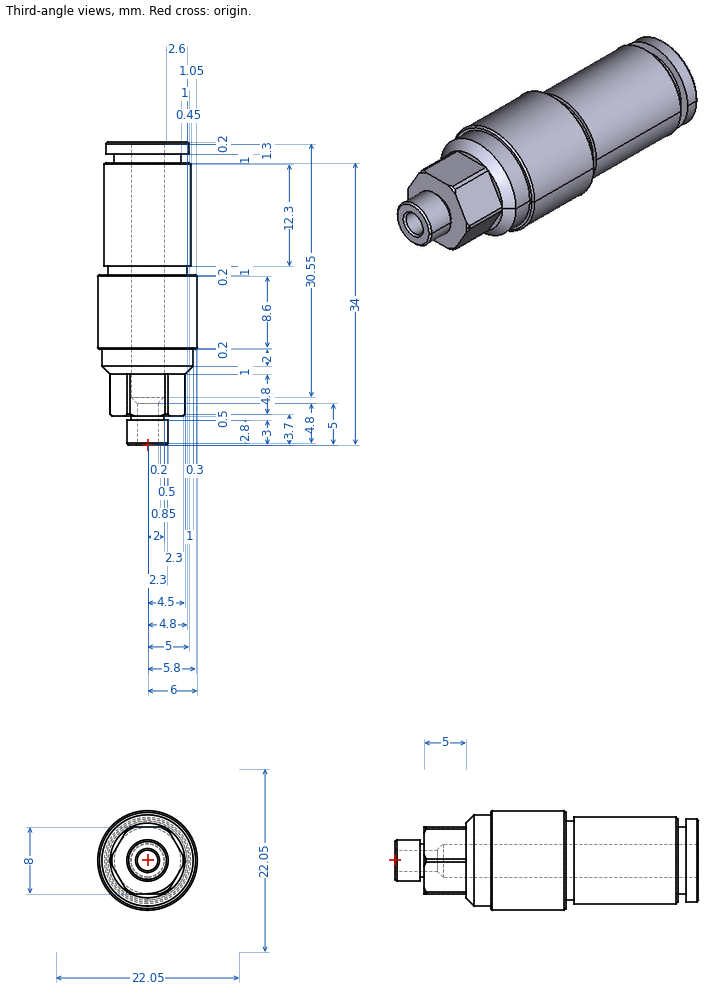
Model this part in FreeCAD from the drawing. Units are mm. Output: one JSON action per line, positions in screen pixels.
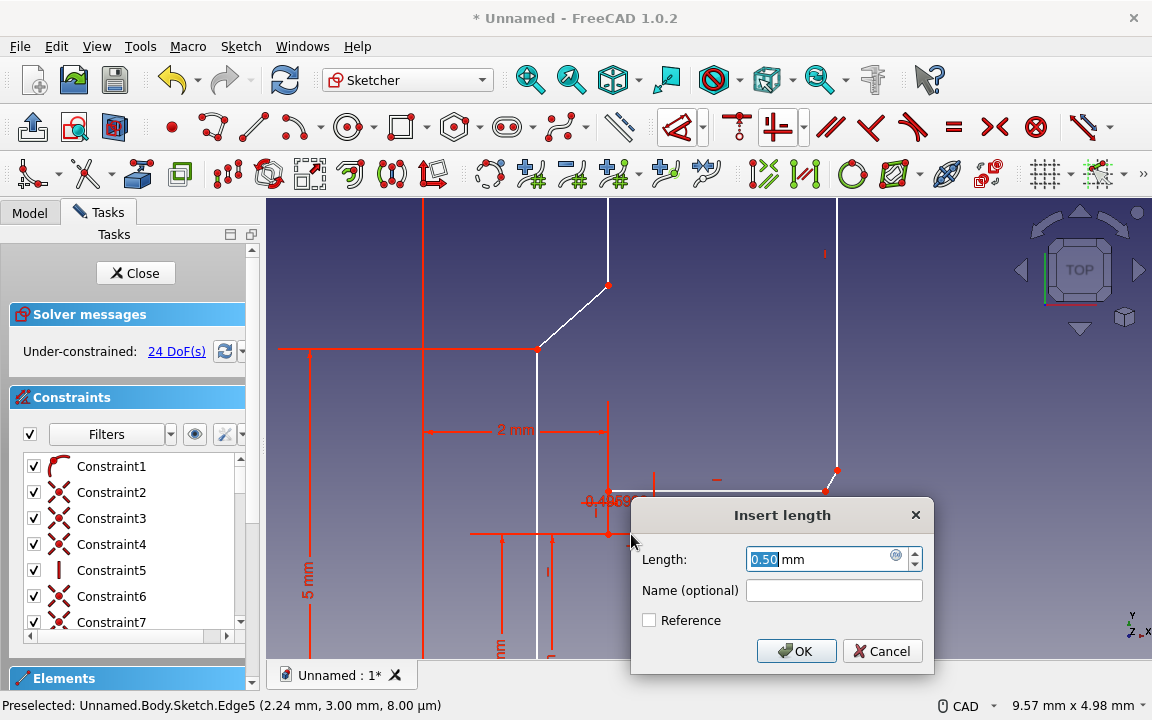
{"action": "type", "text": "0.5"}
{"action": "key", "text": "Return"}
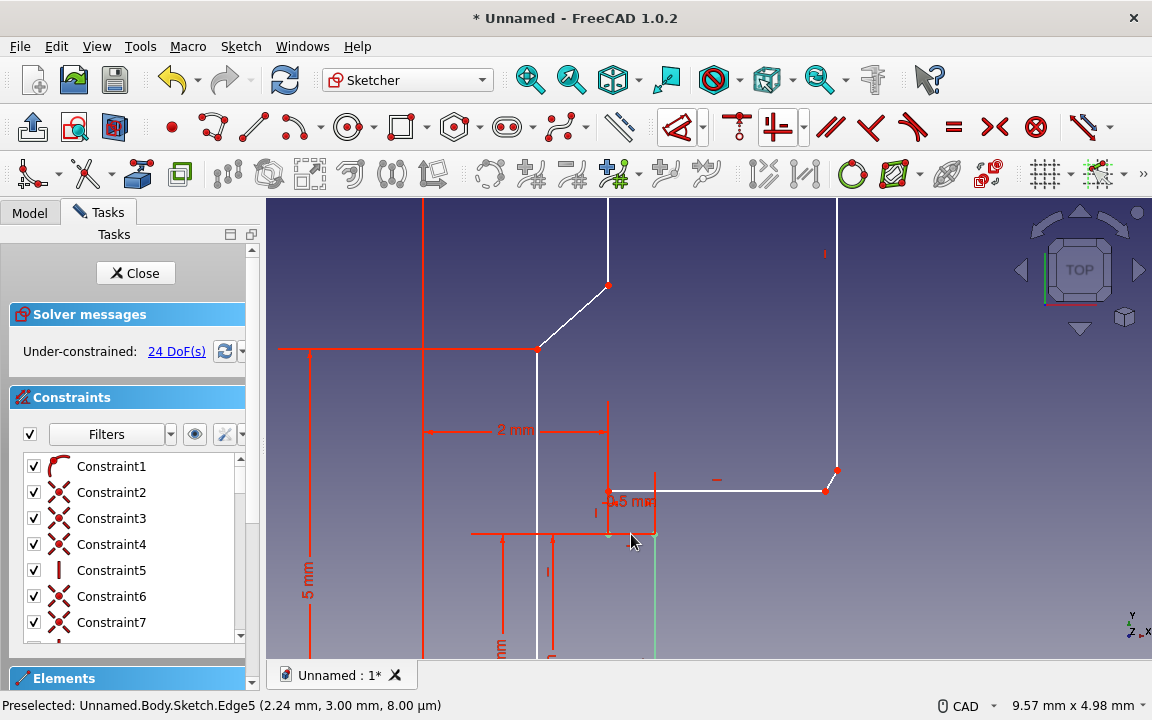
{"action": "left_click", "coordinate": [608, 521]}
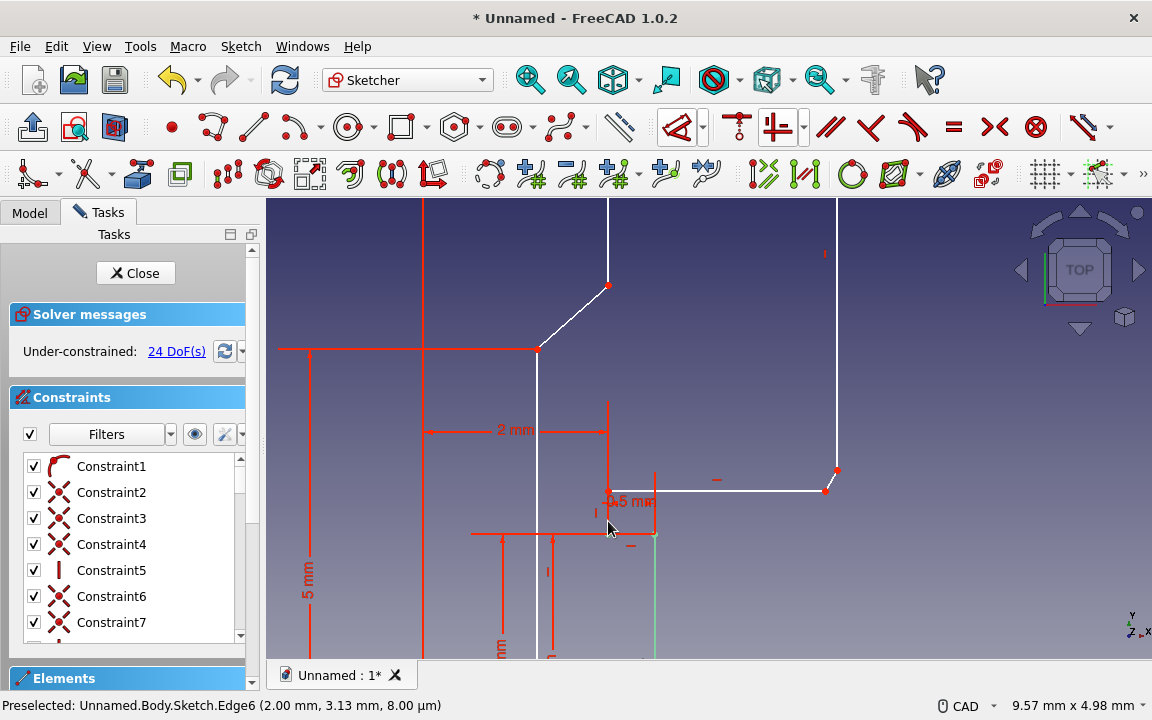
{"action": "left_click", "coordinate": [702, 128]}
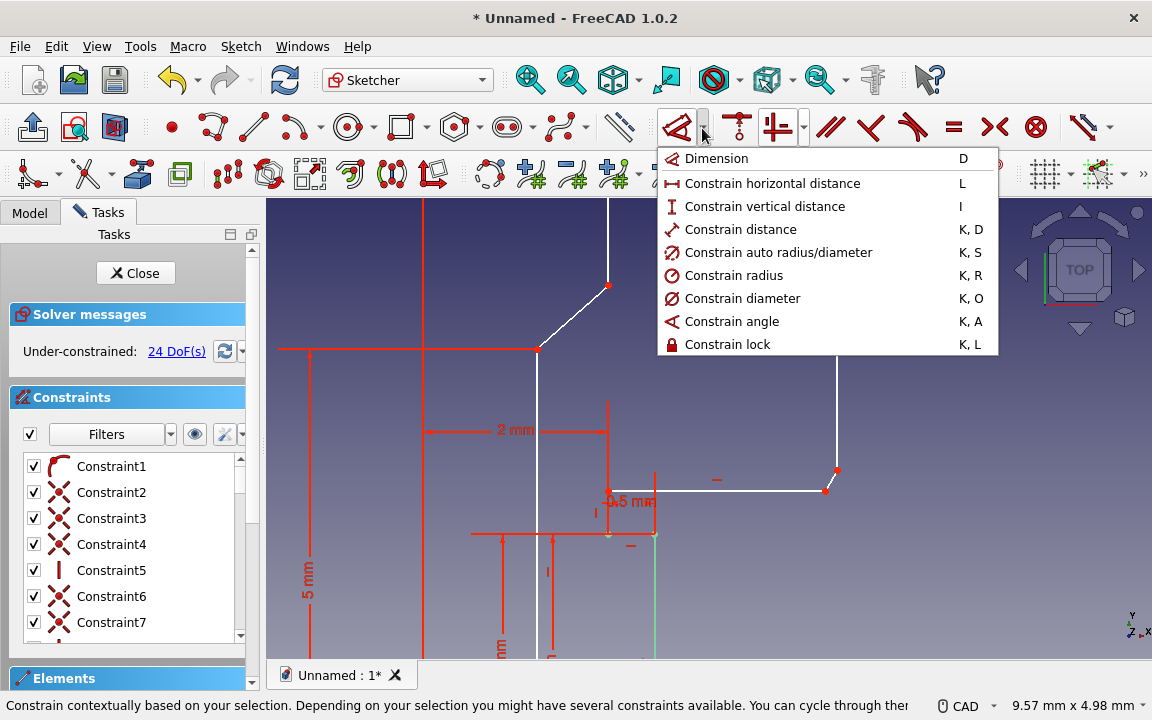
{"action": "left_click", "coordinate": [828, 206]}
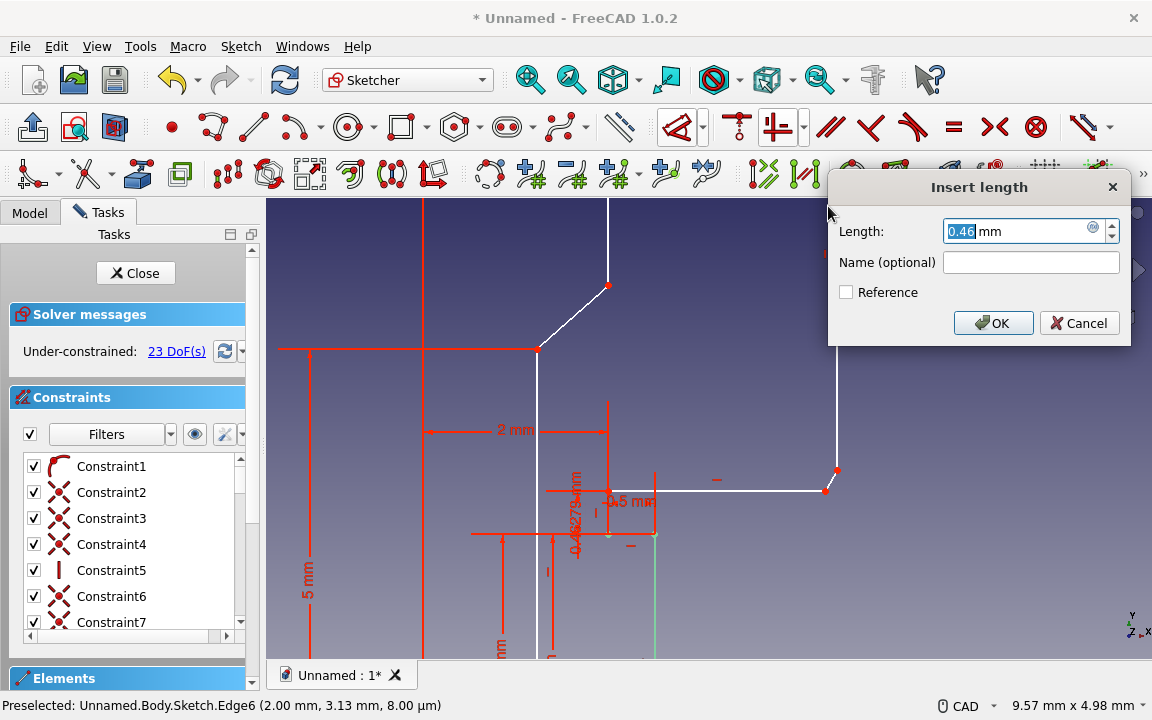
{"action": "type", "text": "0.5"}
{"action": "key", "text": "Return"}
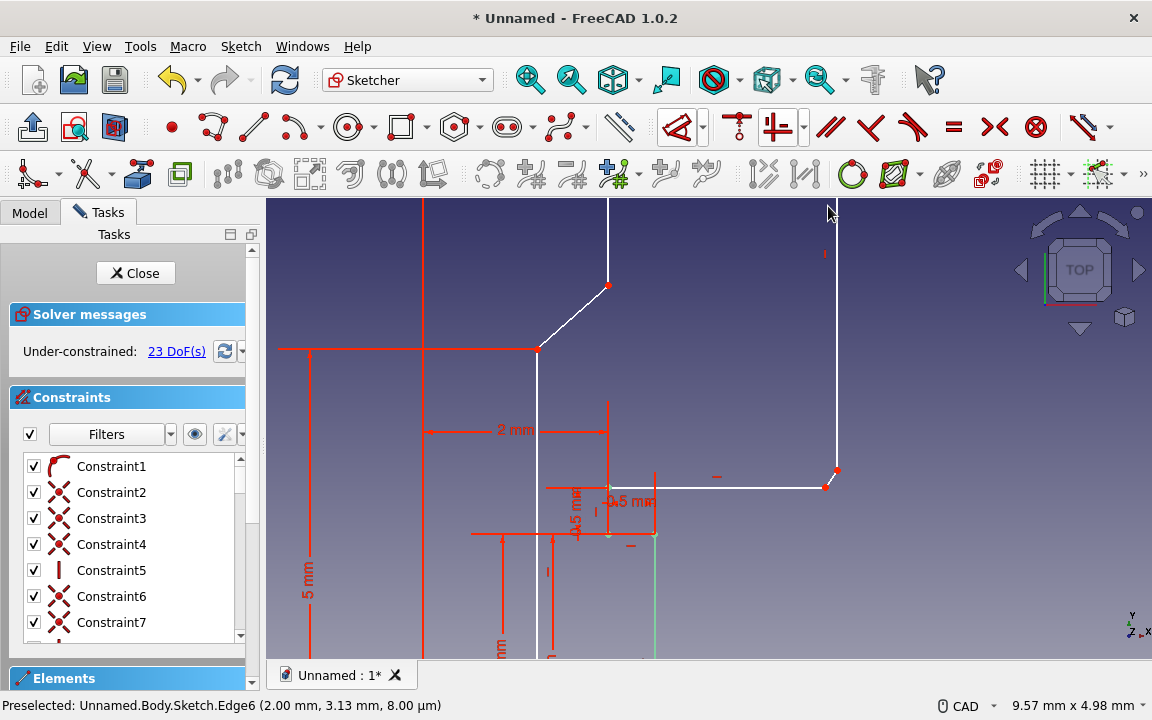
{"action": "scroll", "coordinate": [634, 559], "scroll_direction": "down", "scroll_amount": 12}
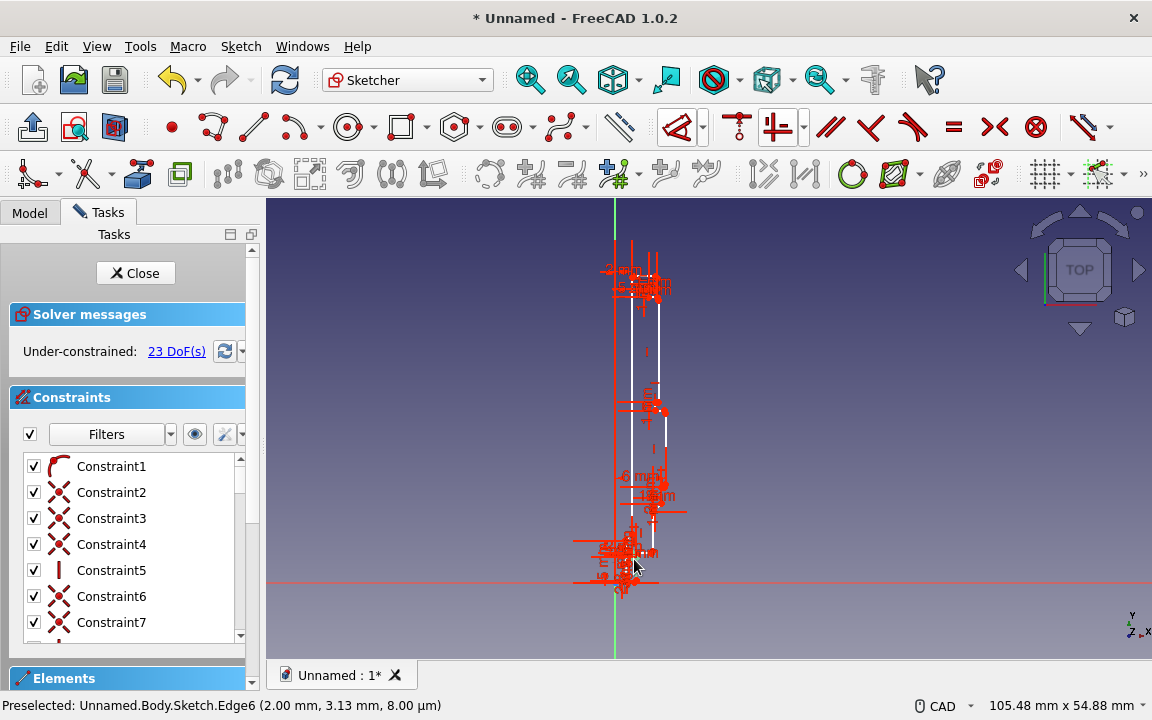
{"action": "scroll", "coordinate": [638, 553], "scroll_direction": "up", "scroll_amount": 6}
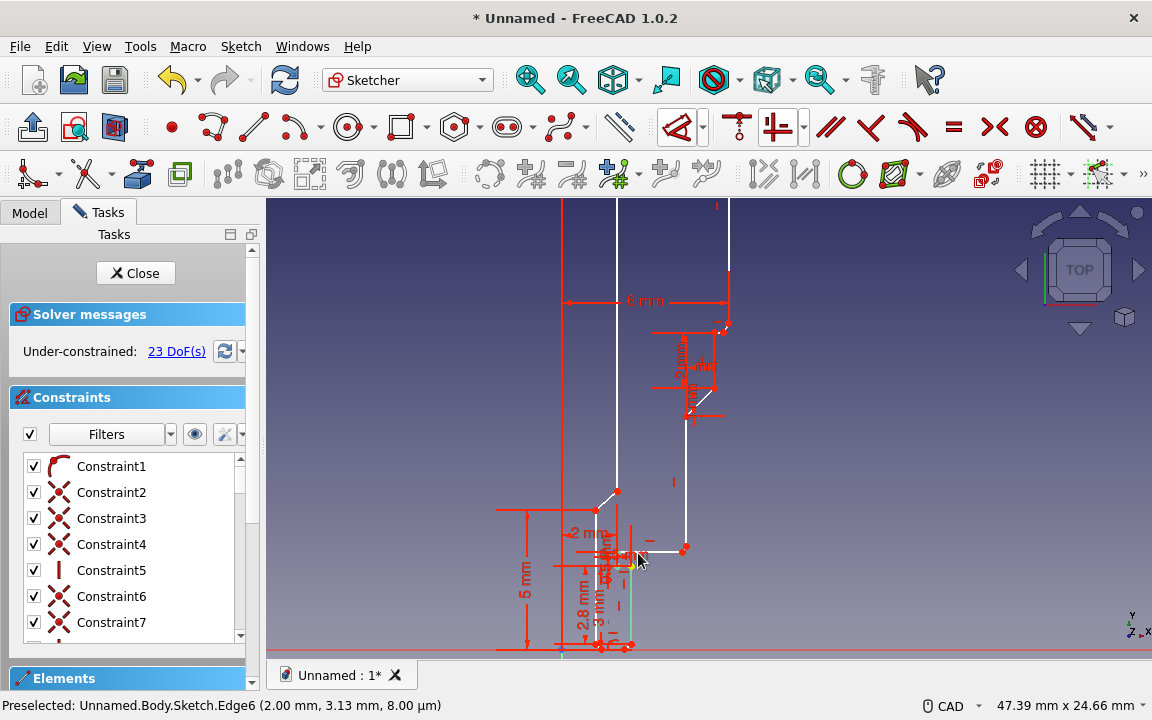
{"action": "left_click", "coordinate": [663, 552]}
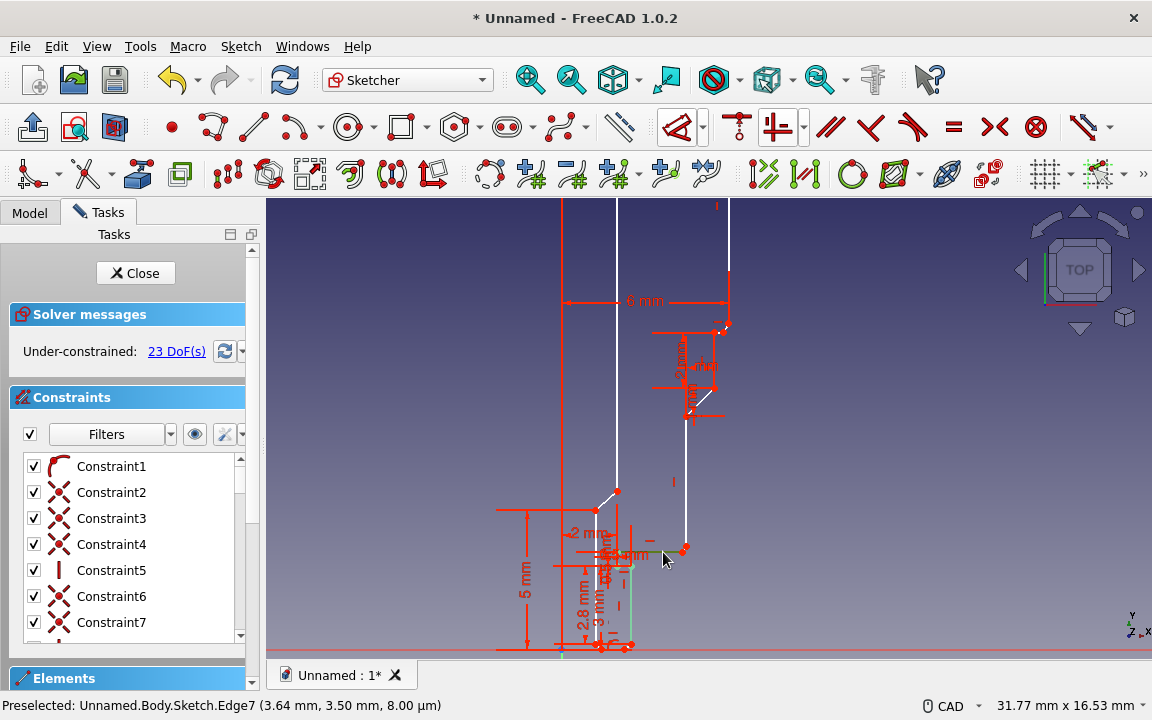
{"action": "left_click", "coordinate": [702, 128]}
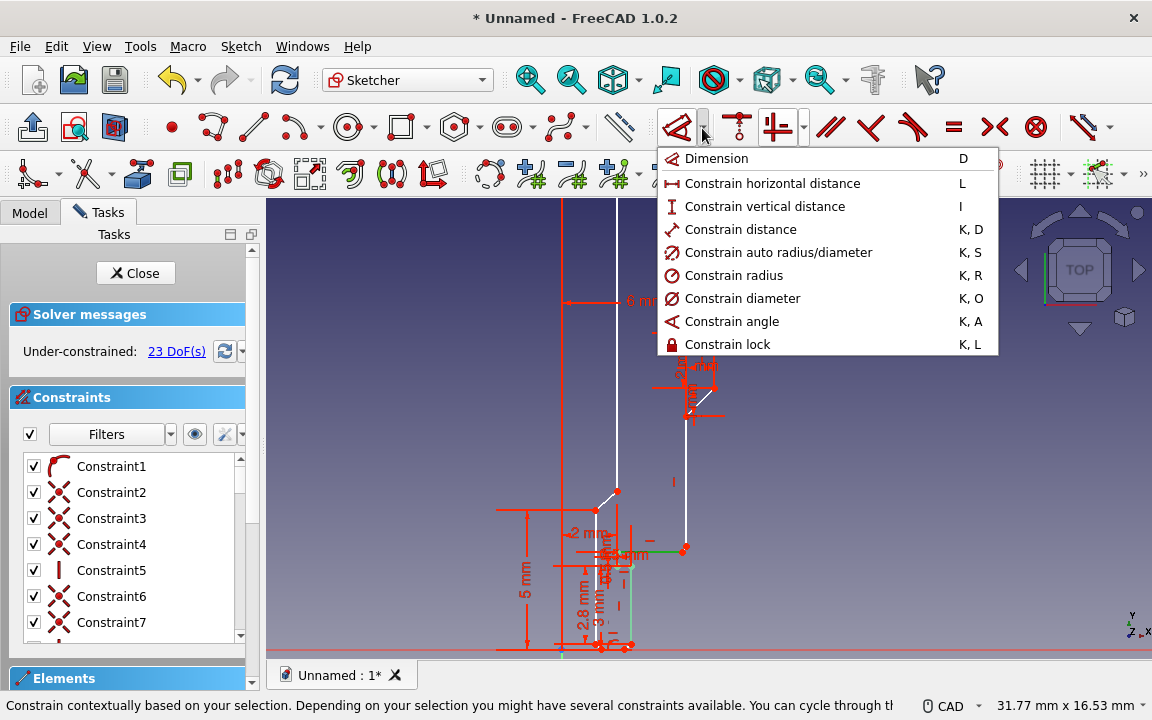
{"action": "left_click", "coordinate": [828, 184]}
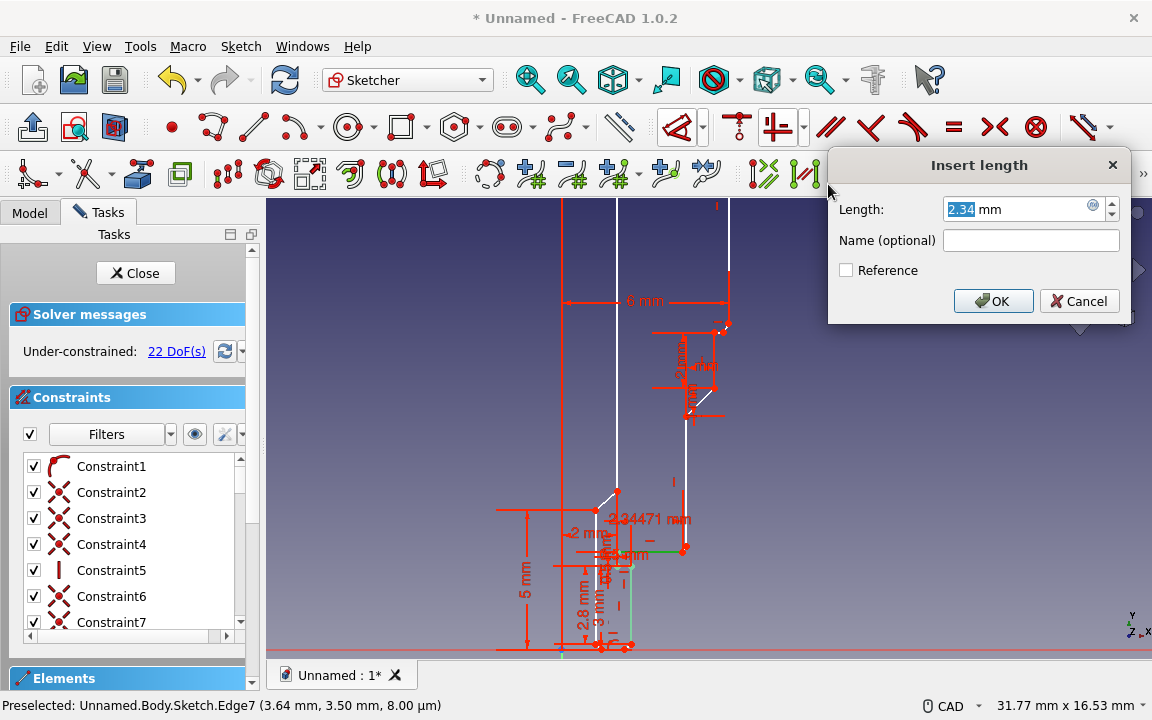
{"action": "type", "text": "2.3"}
{"action": "key", "text": "Return"}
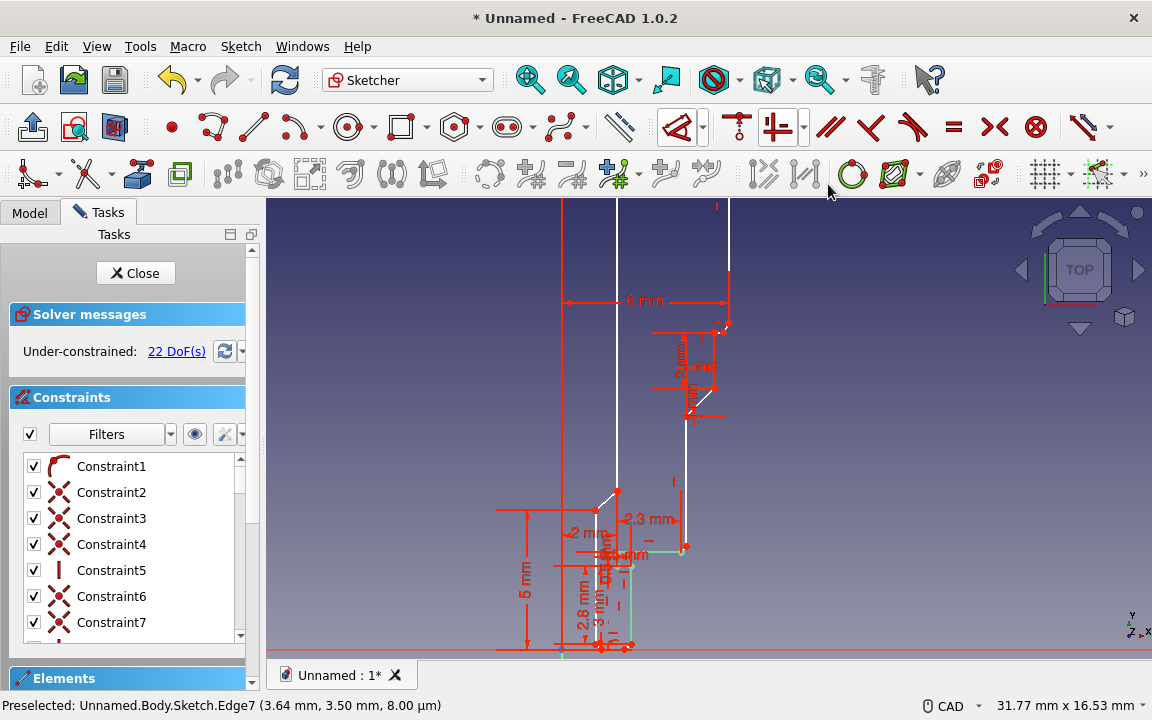
{"action": "left_click", "coordinate": [686, 508]}